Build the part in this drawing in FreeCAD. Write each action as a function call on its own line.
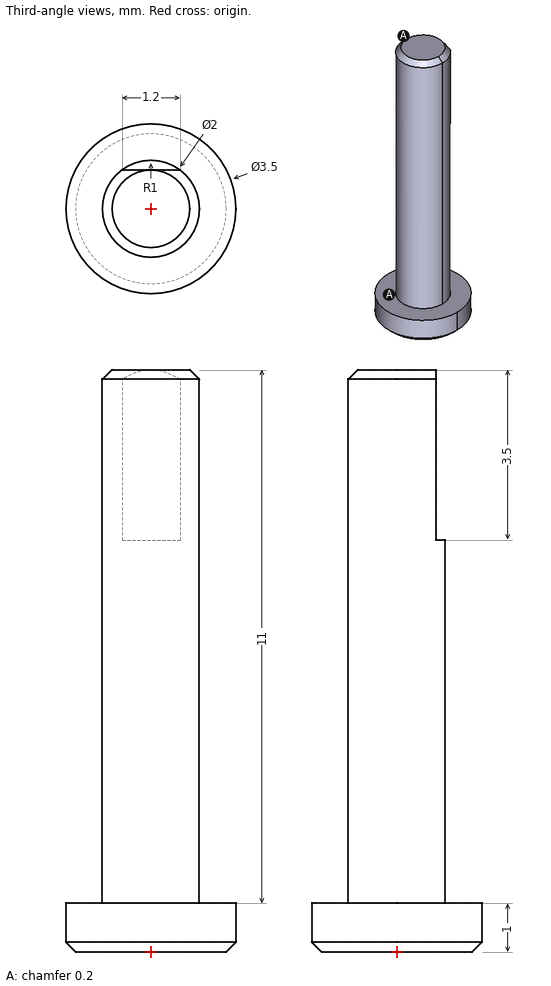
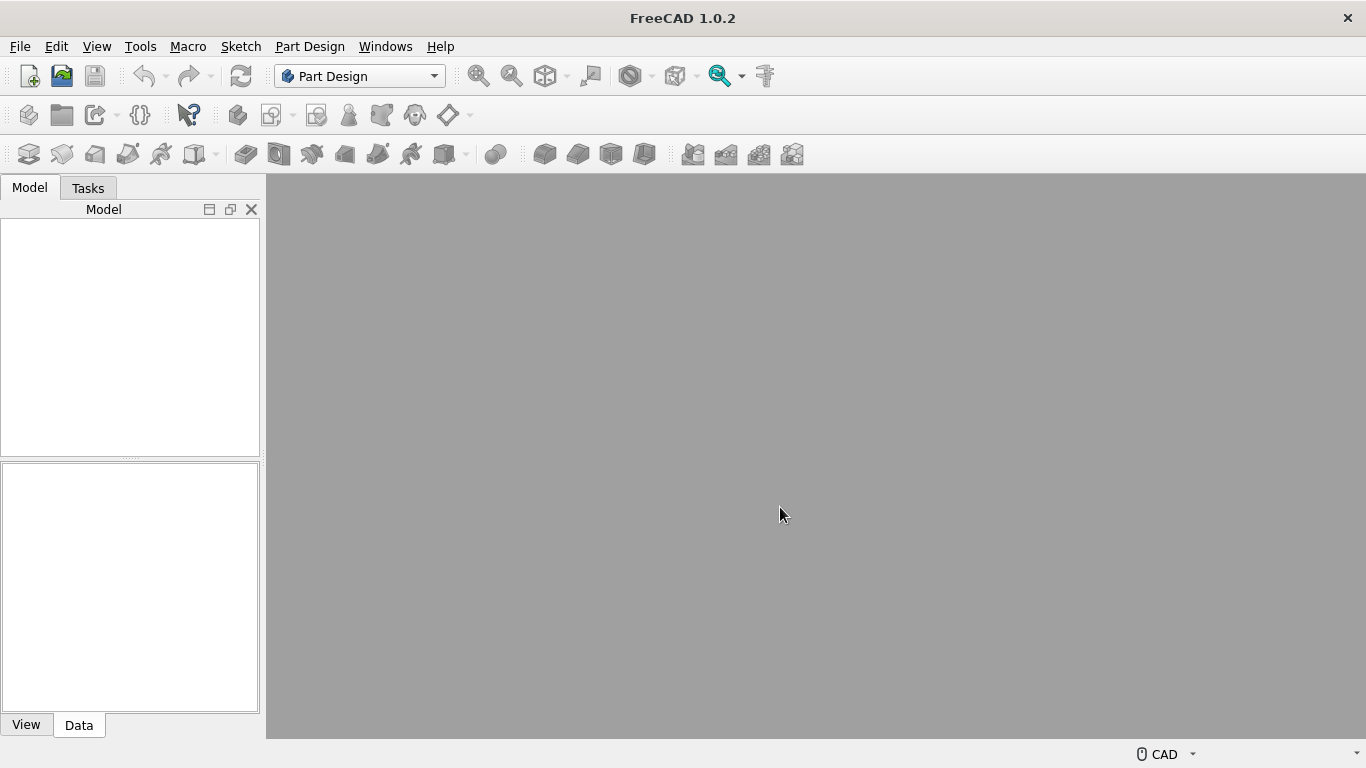
click(29, 76)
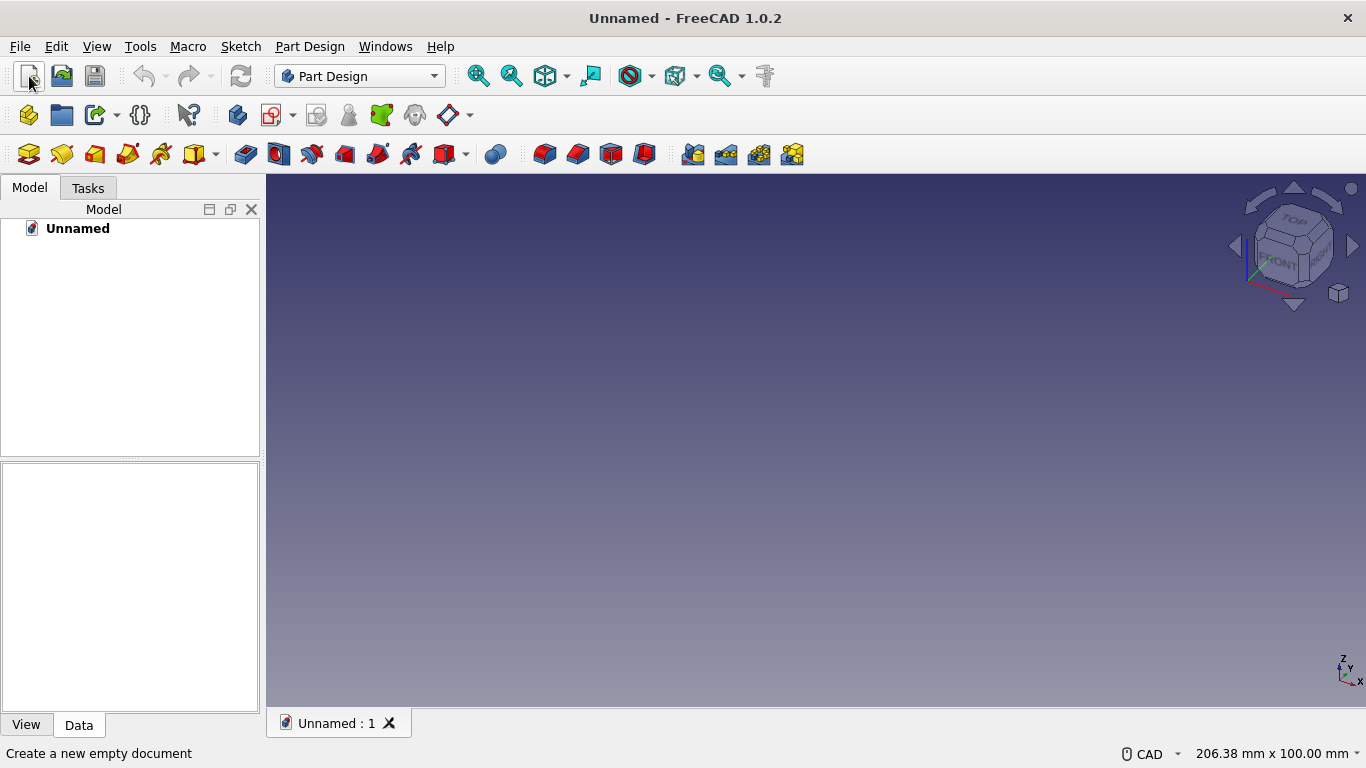
click(270, 116)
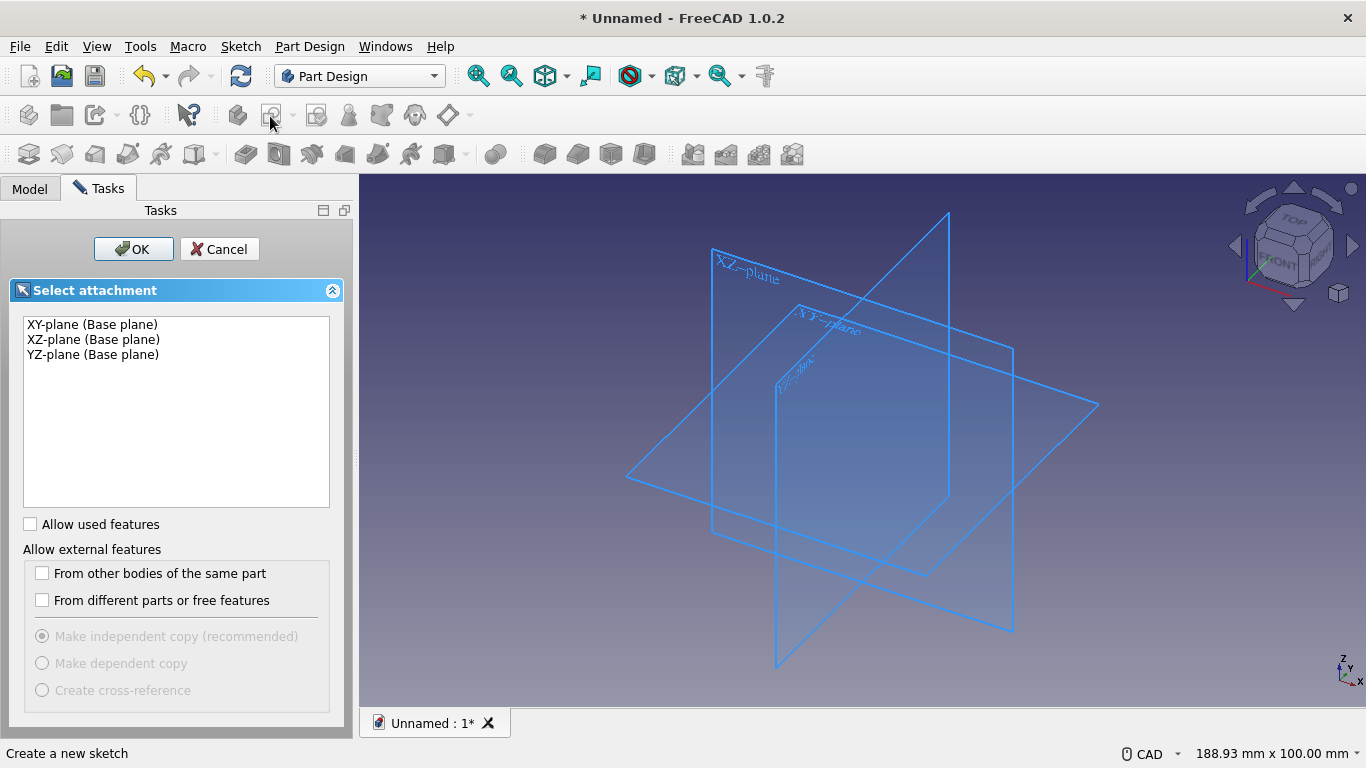
click(84, 324)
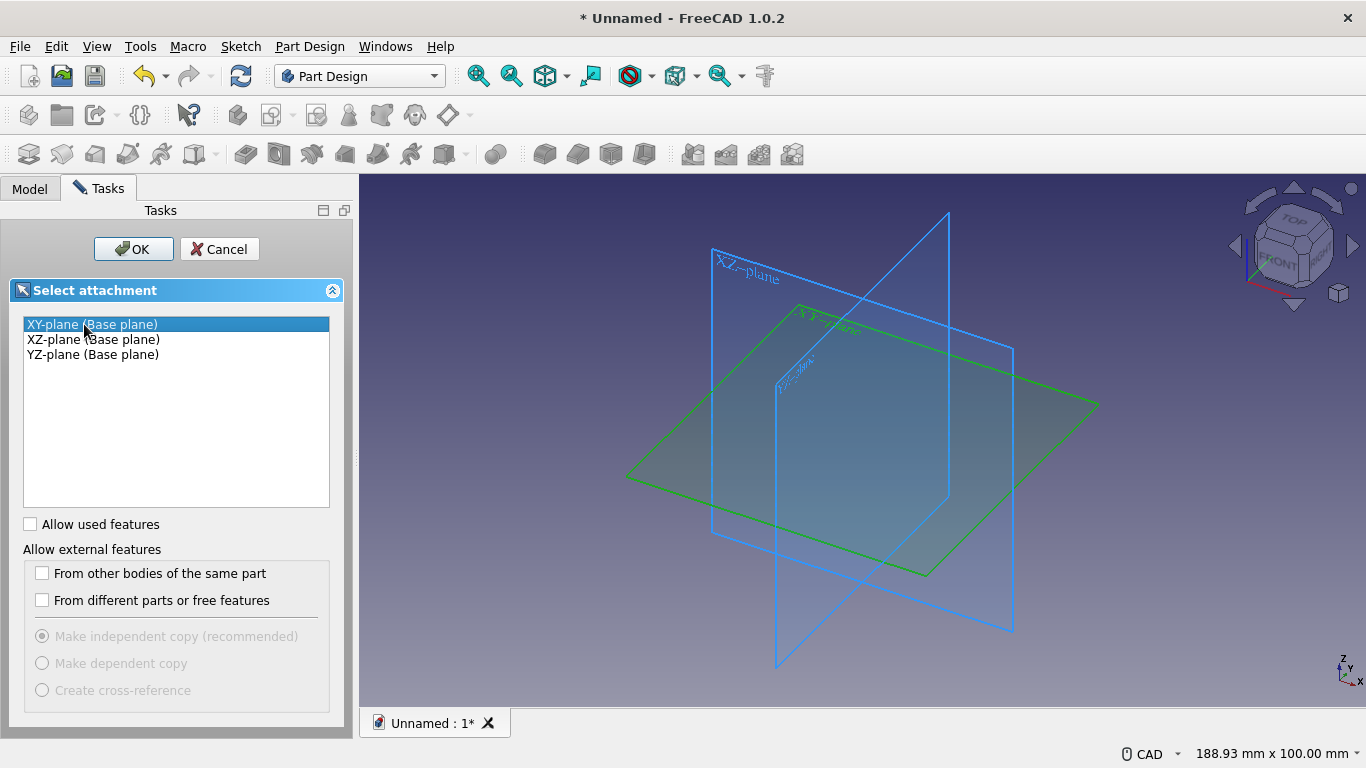
click(134, 249)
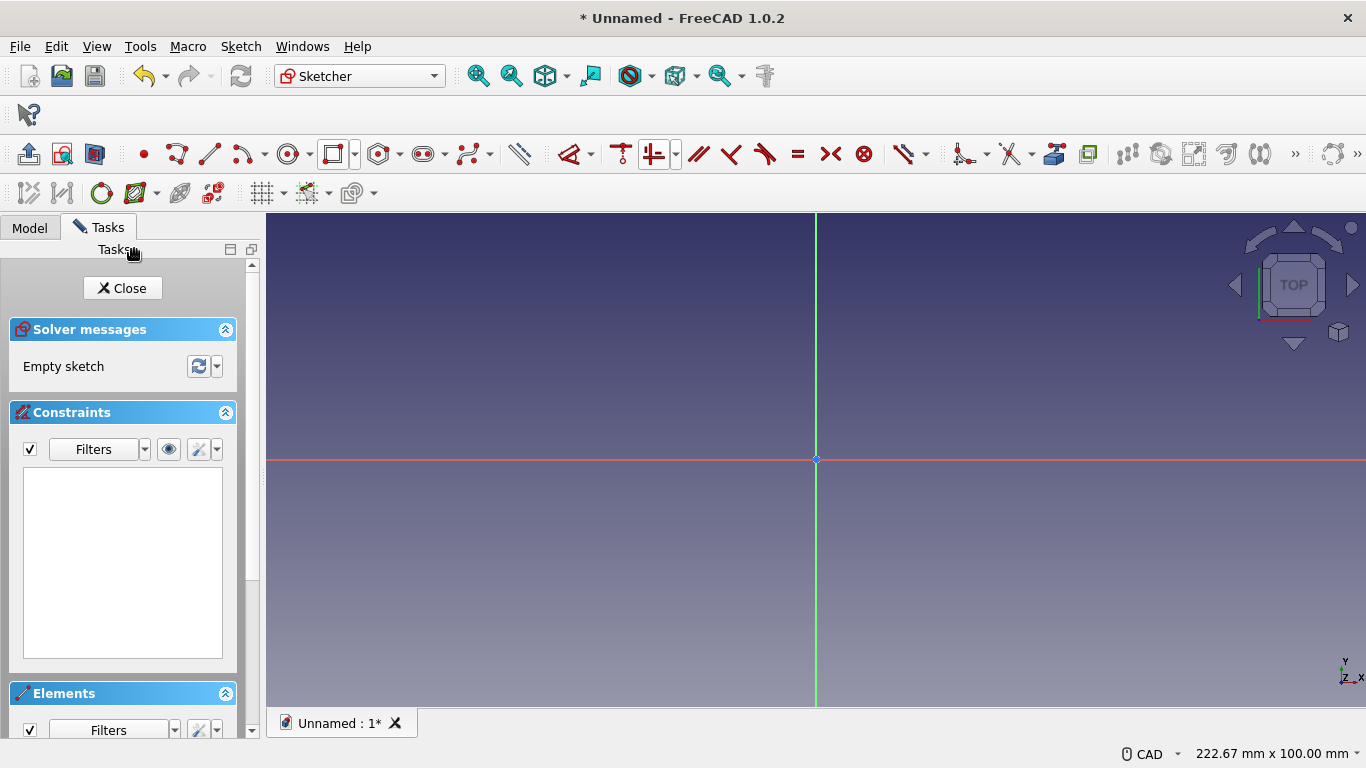
scroll(820, 460, up, 14)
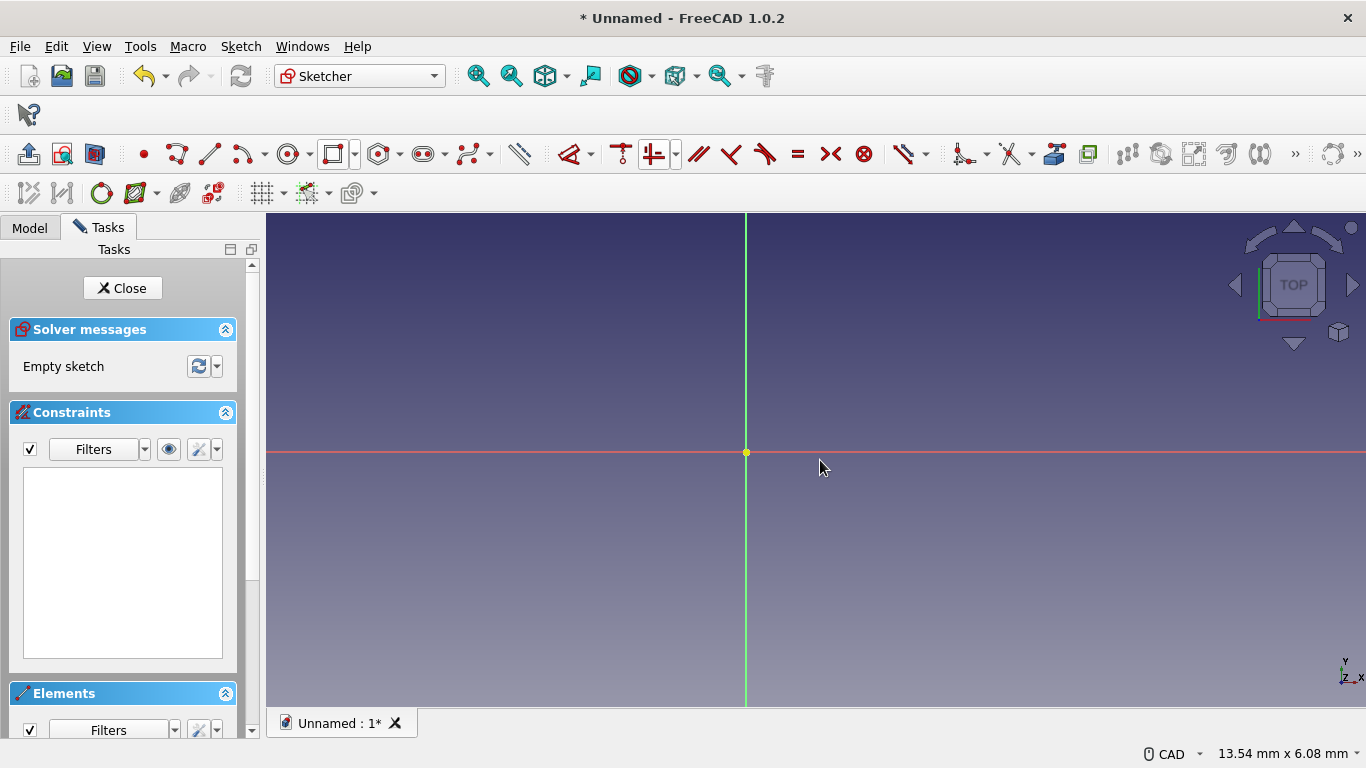
click(288, 154)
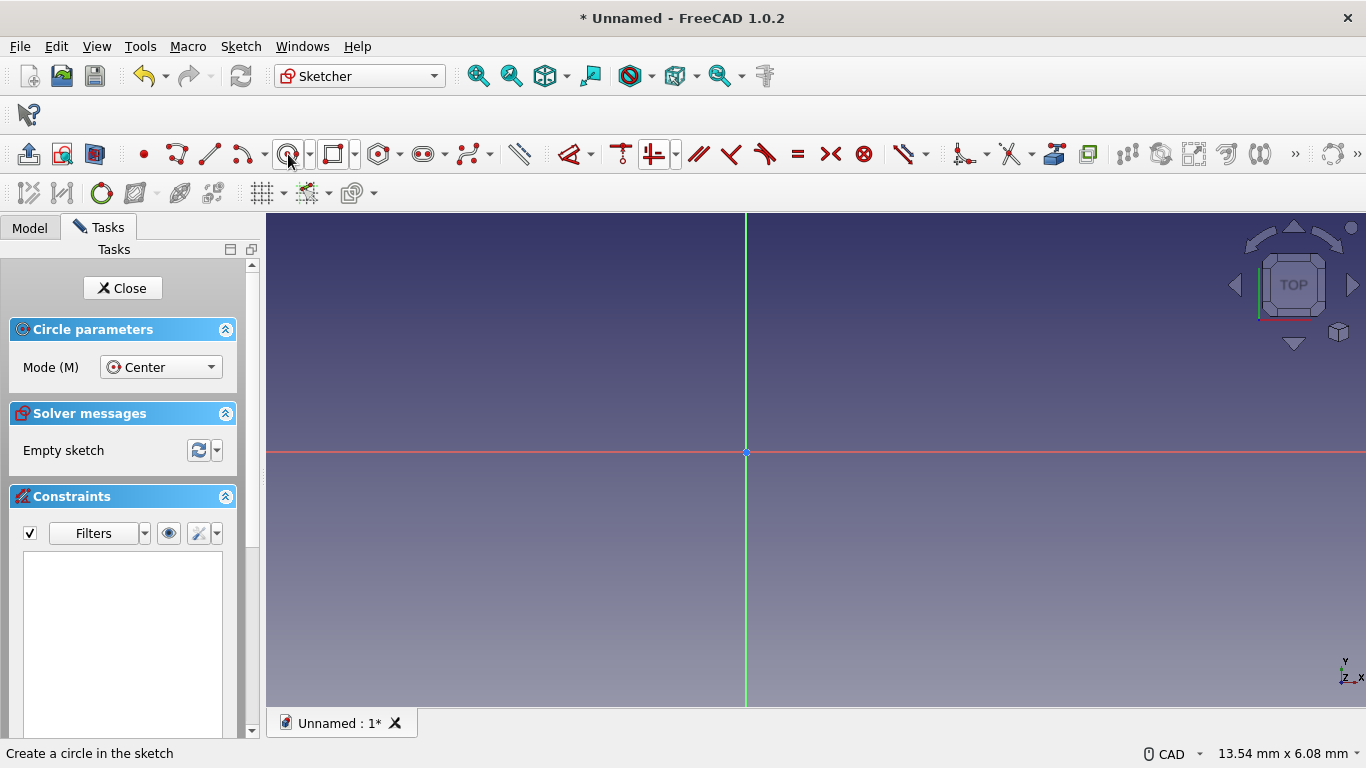
click(746, 452)
move(847, 352)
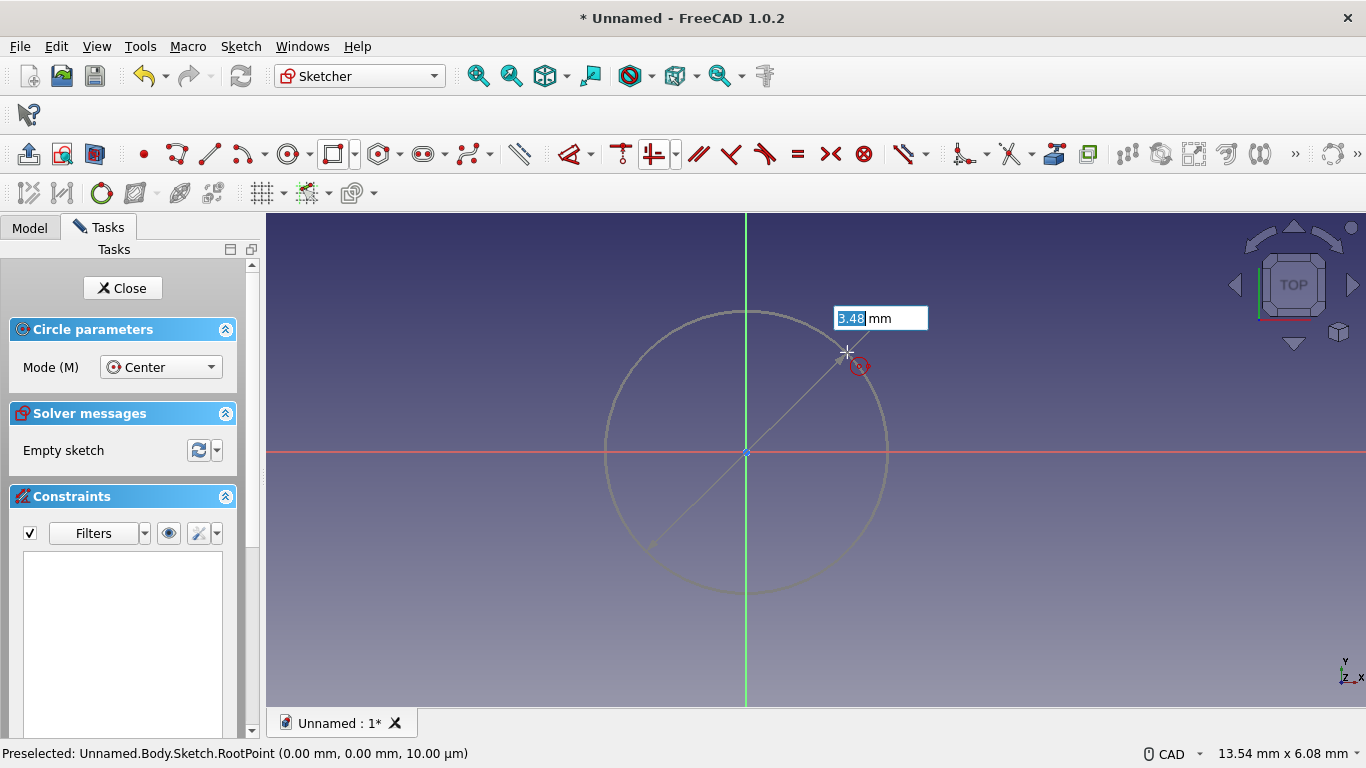
text(3.5)
key(Return)
key(Escape)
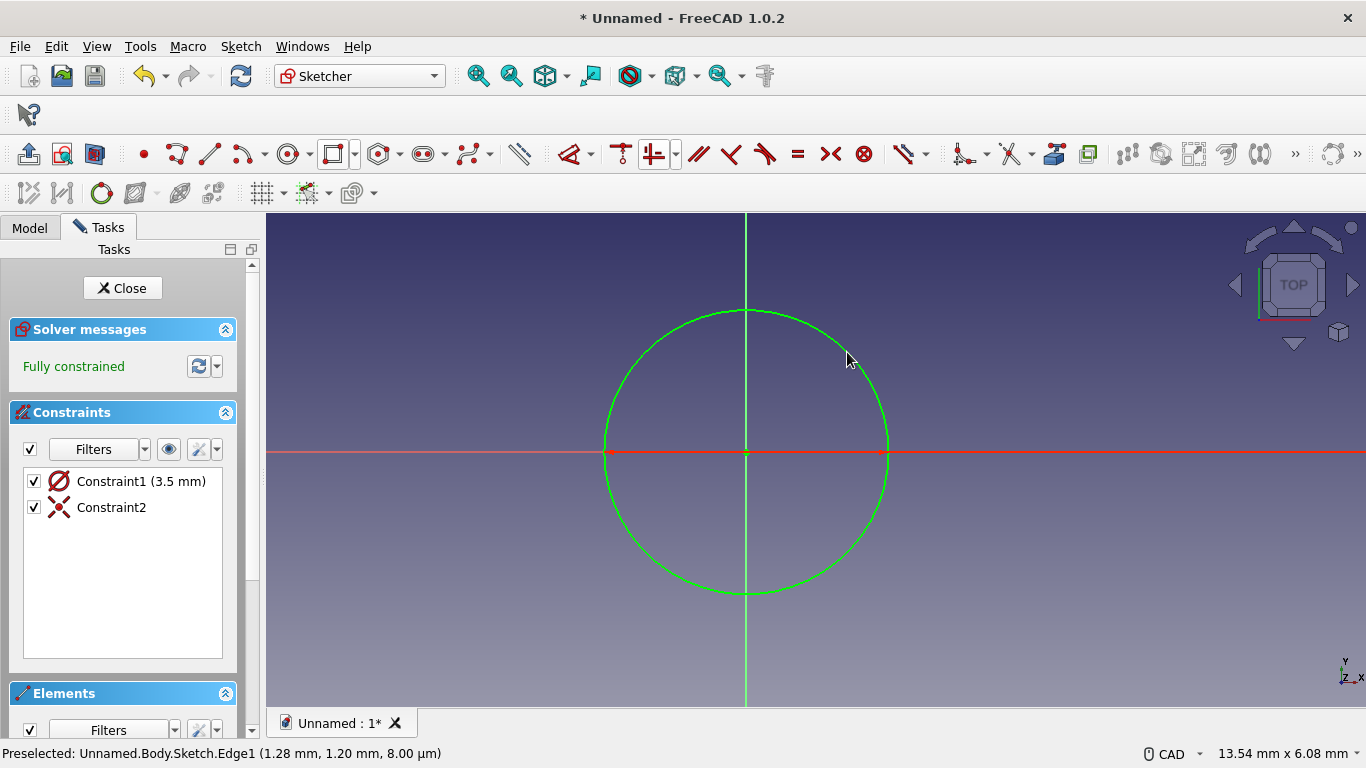
click(123, 288)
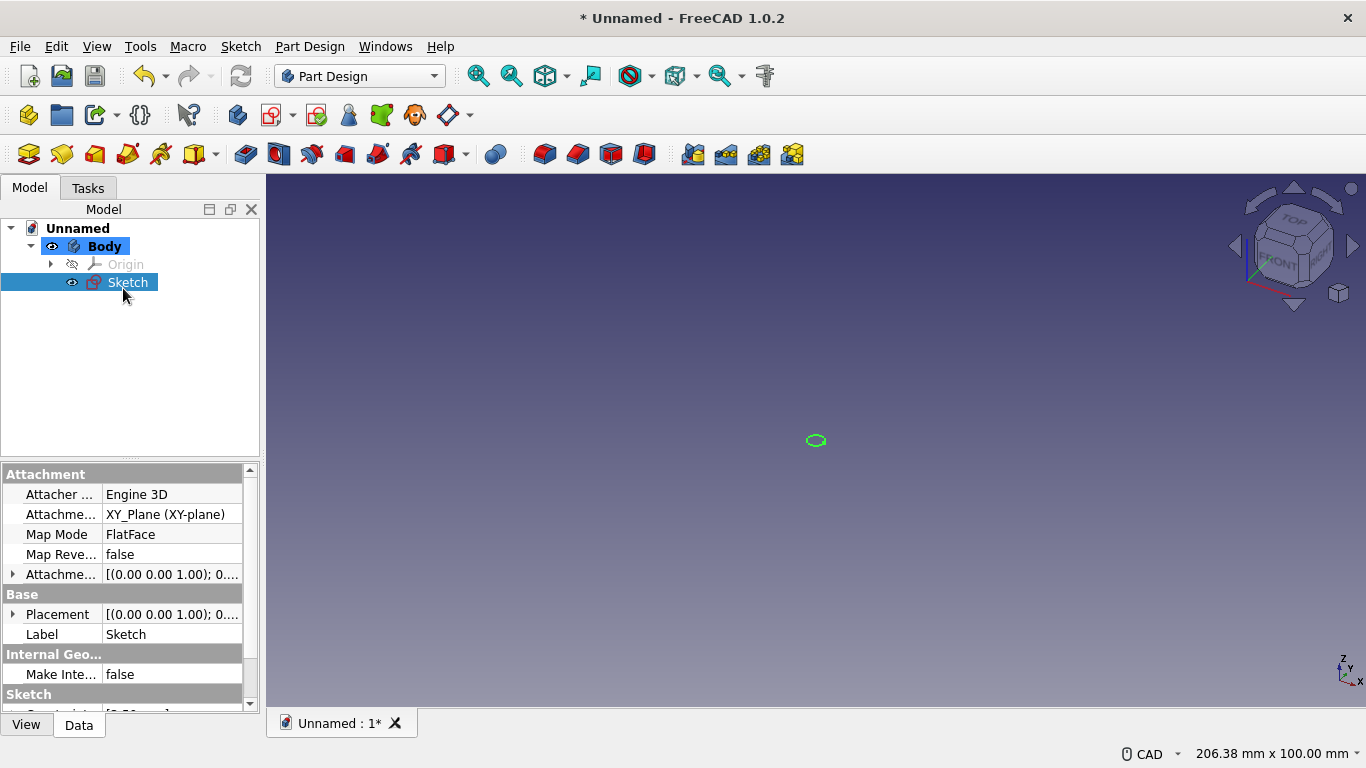
click(29, 154)